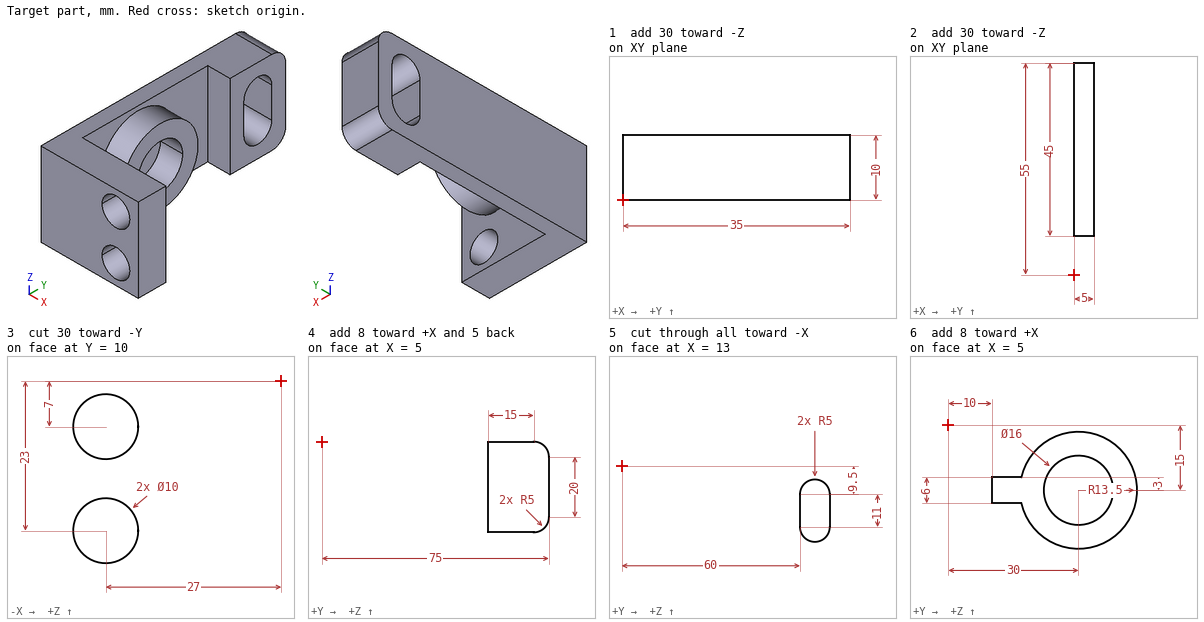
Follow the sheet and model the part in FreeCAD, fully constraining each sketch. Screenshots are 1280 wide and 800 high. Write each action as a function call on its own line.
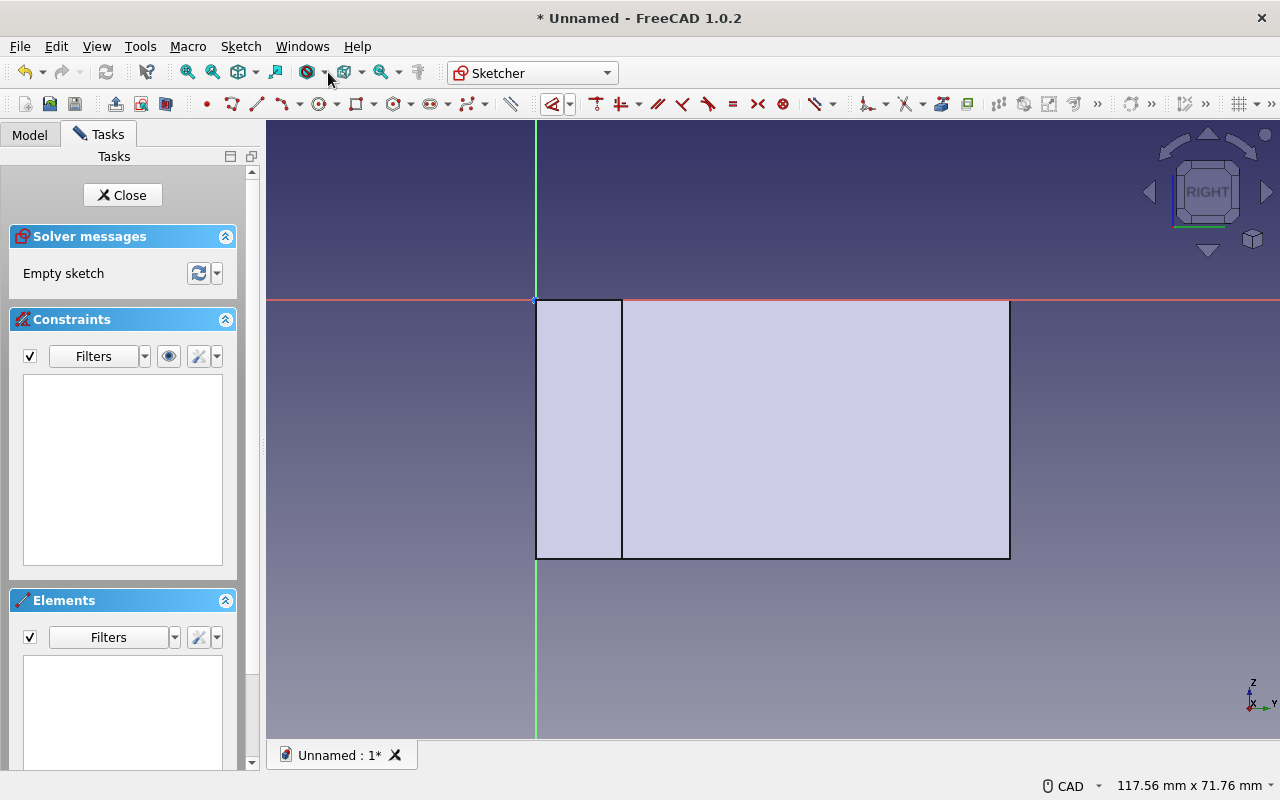
scroll(294, 430, down, 1)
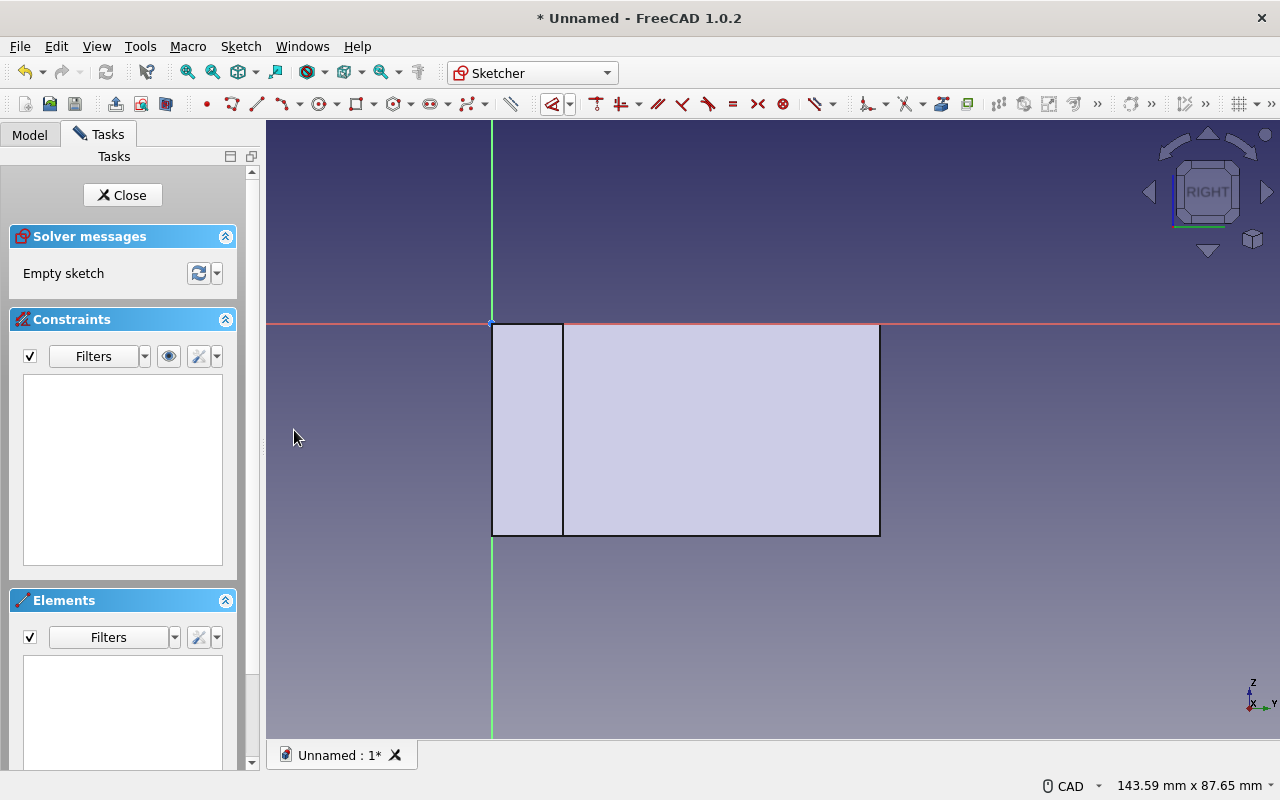
scroll(1115, 430, up, 3)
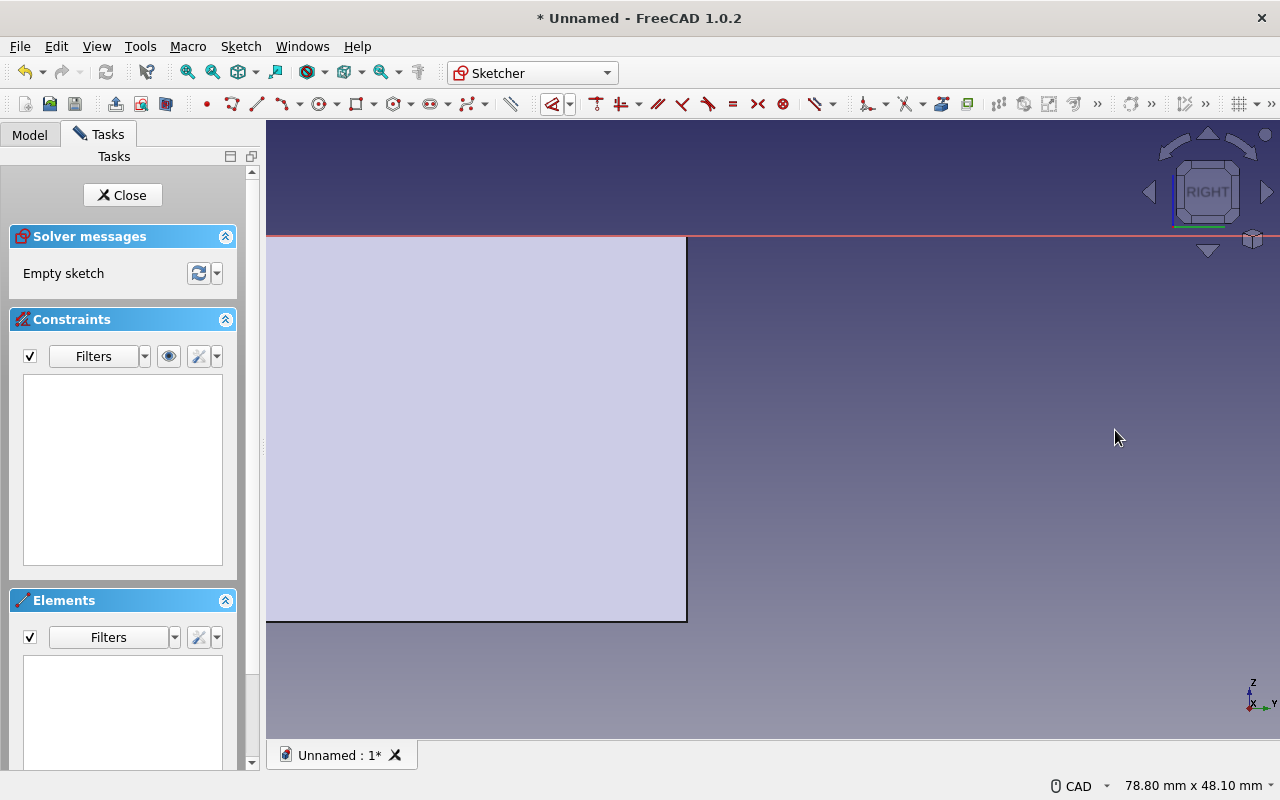
key(g)
key(l)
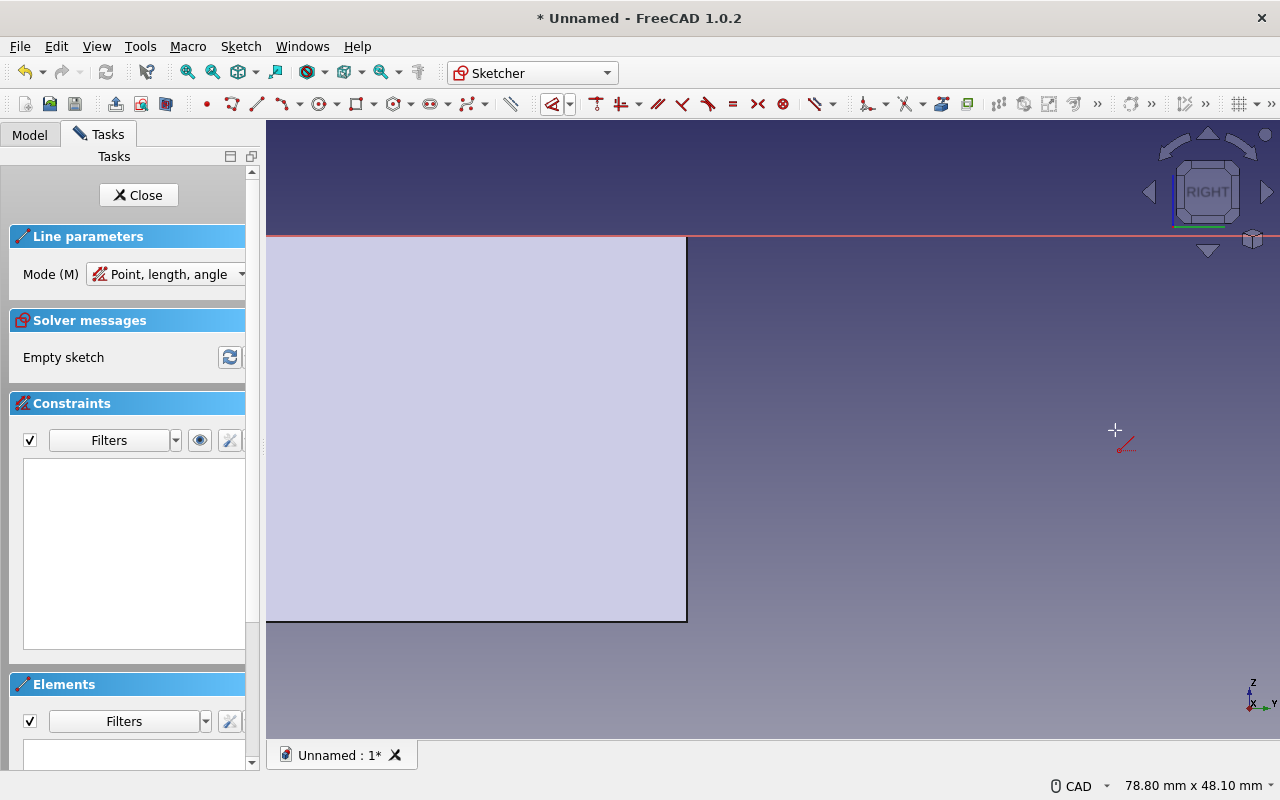
click(944, 558)
click(944, 300)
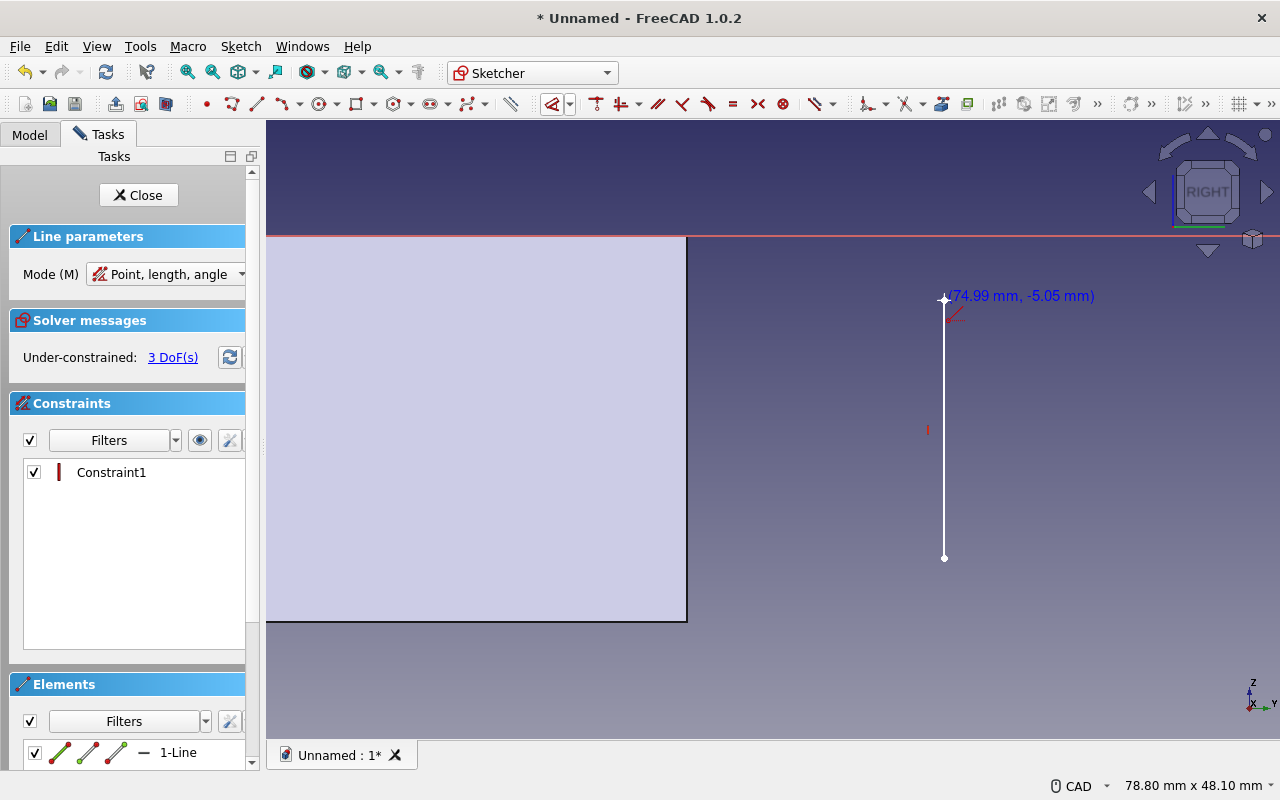
key(g)
key(m)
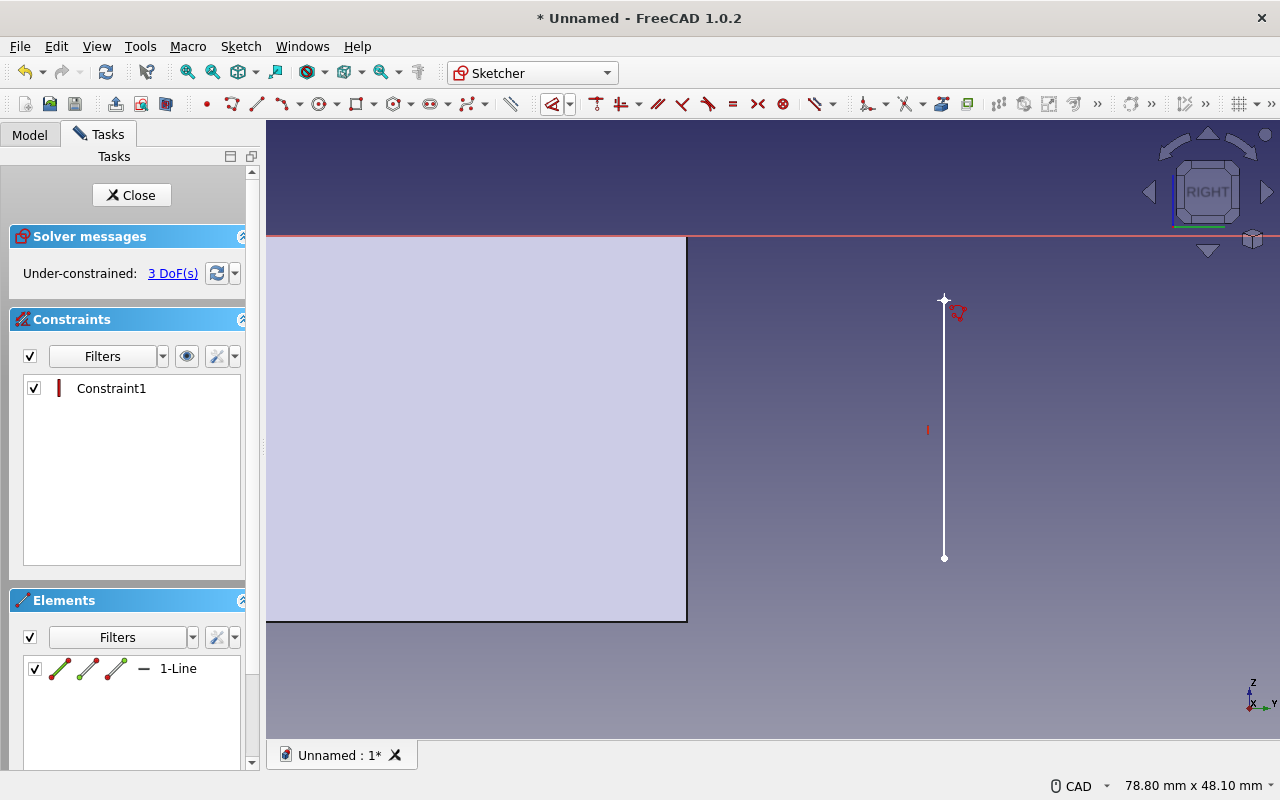
click(880, 236)
click(687, 245)
click(687, 622)
click(880, 622)
right_click(880, 622)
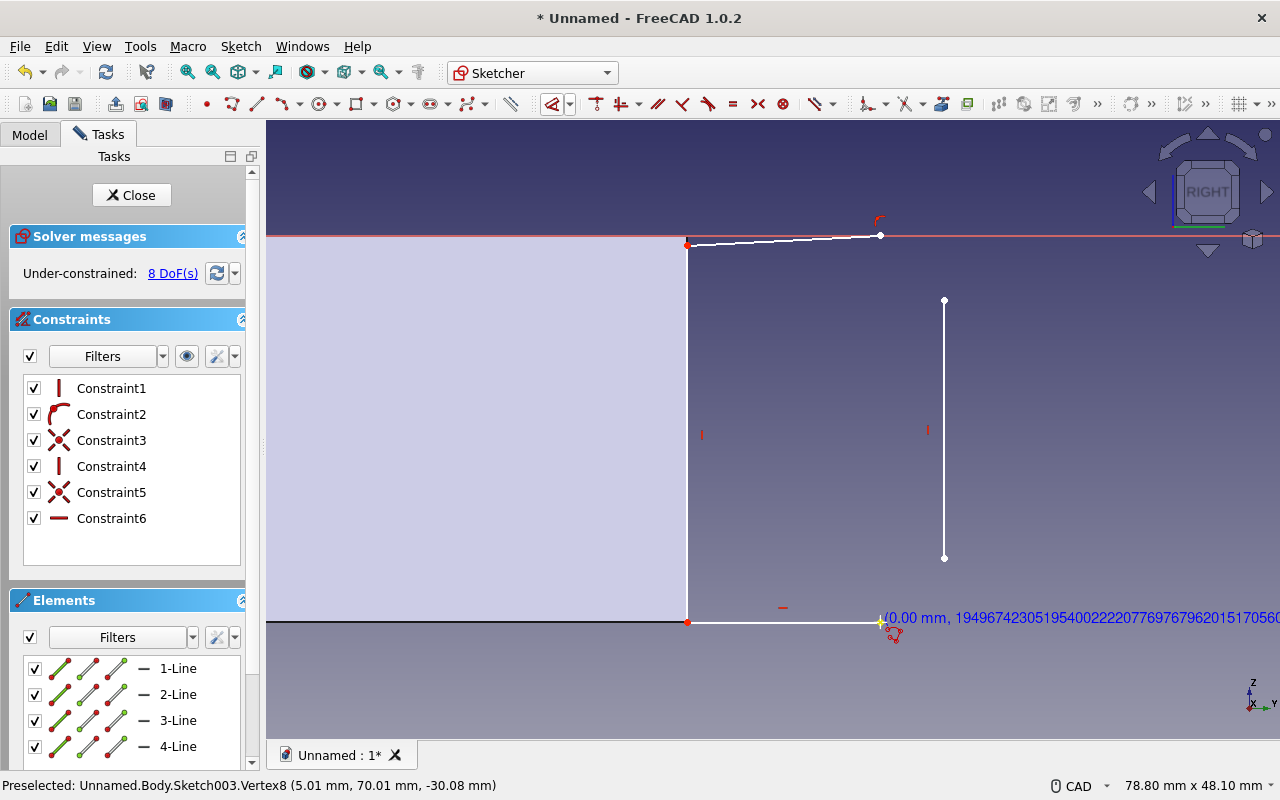
key(g)
key(3)
key(a)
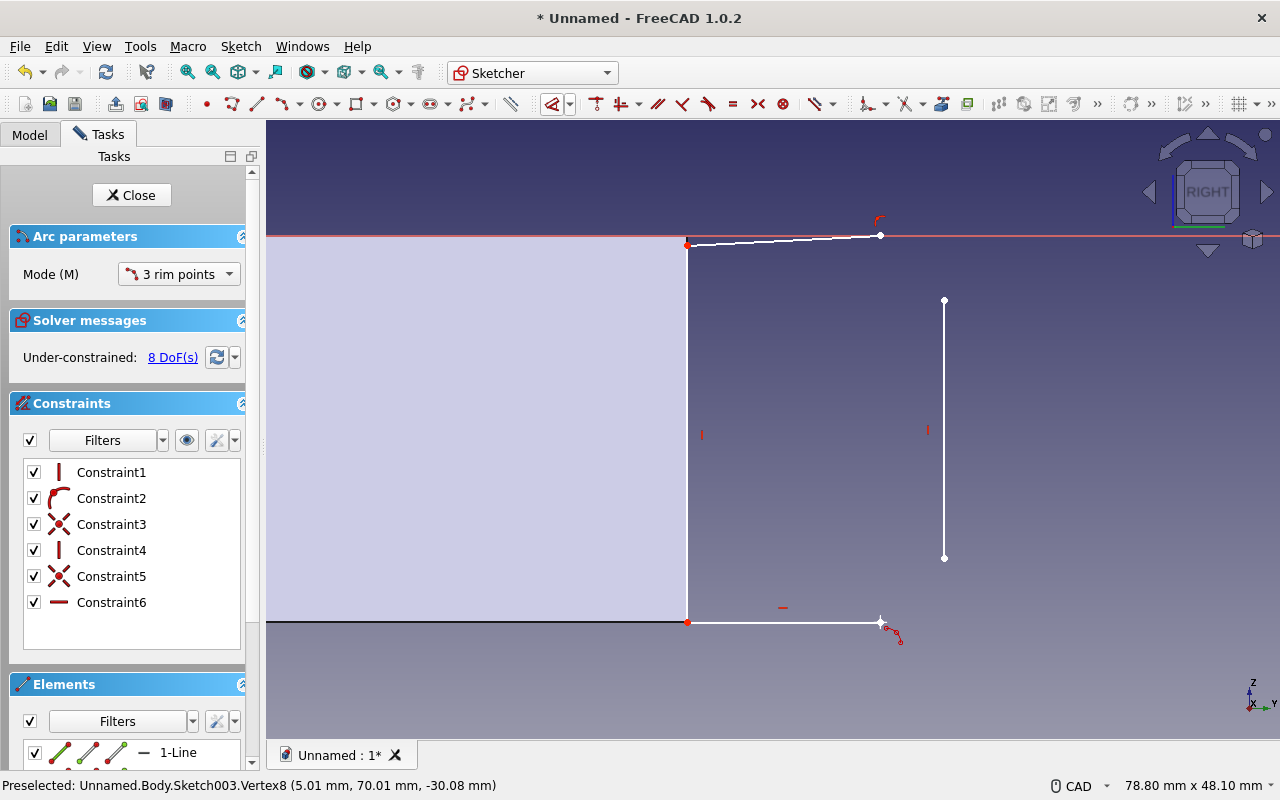
click(944, 301)
click(880, 236)
click(925, 255)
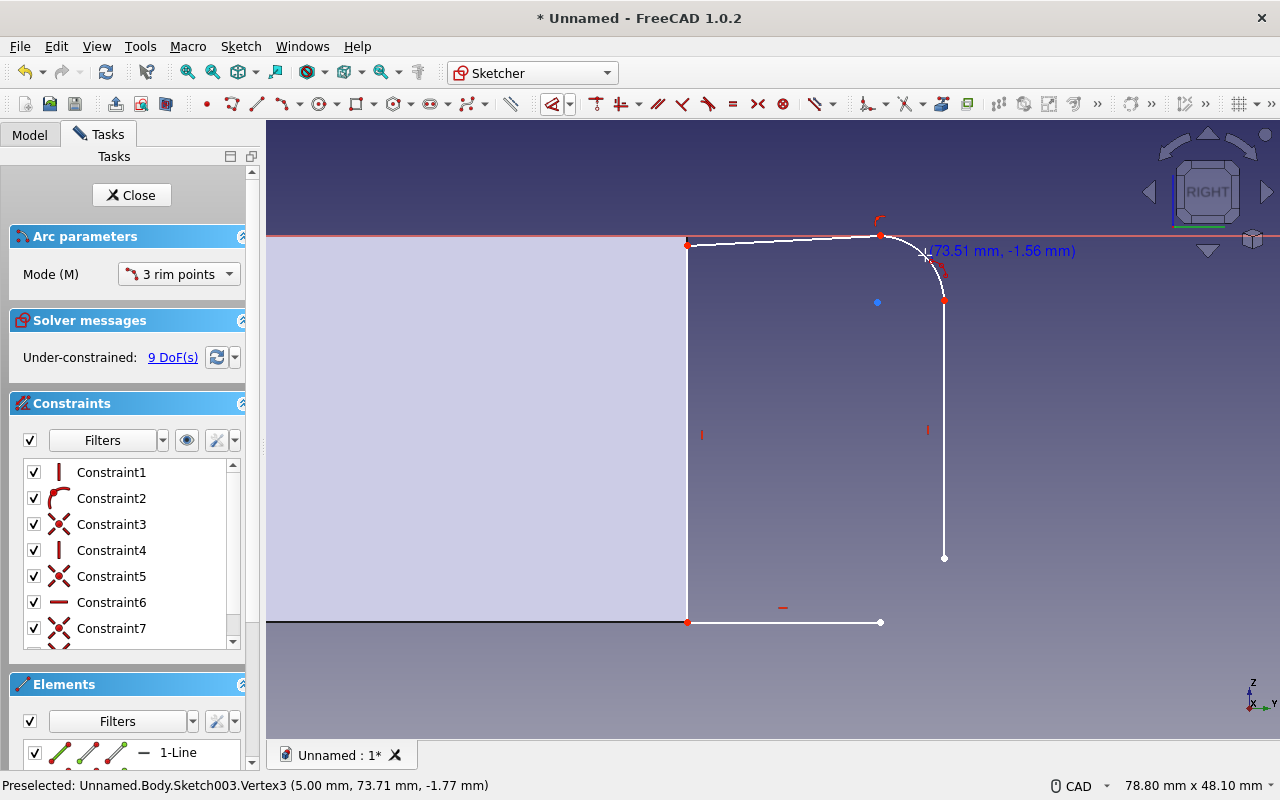
click(880, 623)
click(944, 559)
click(925, 603)
key(Escape)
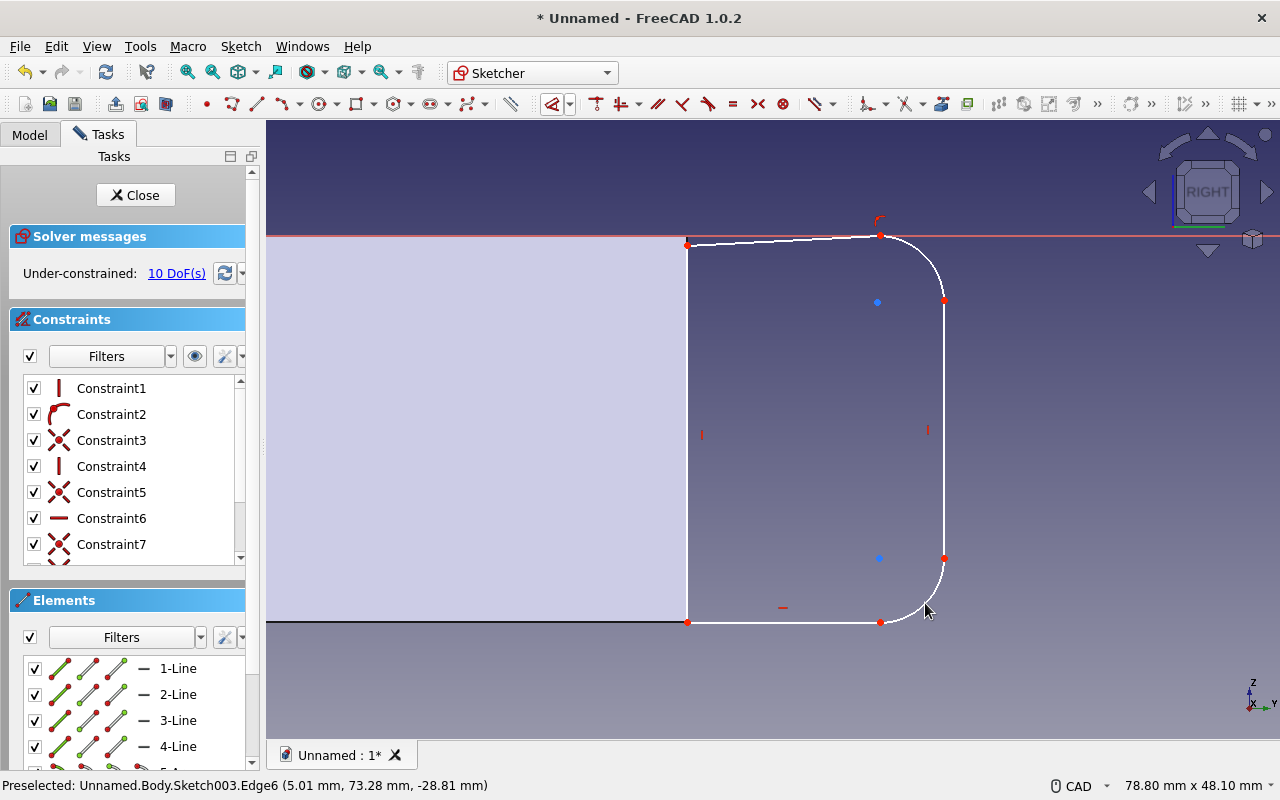
click(944, 482)